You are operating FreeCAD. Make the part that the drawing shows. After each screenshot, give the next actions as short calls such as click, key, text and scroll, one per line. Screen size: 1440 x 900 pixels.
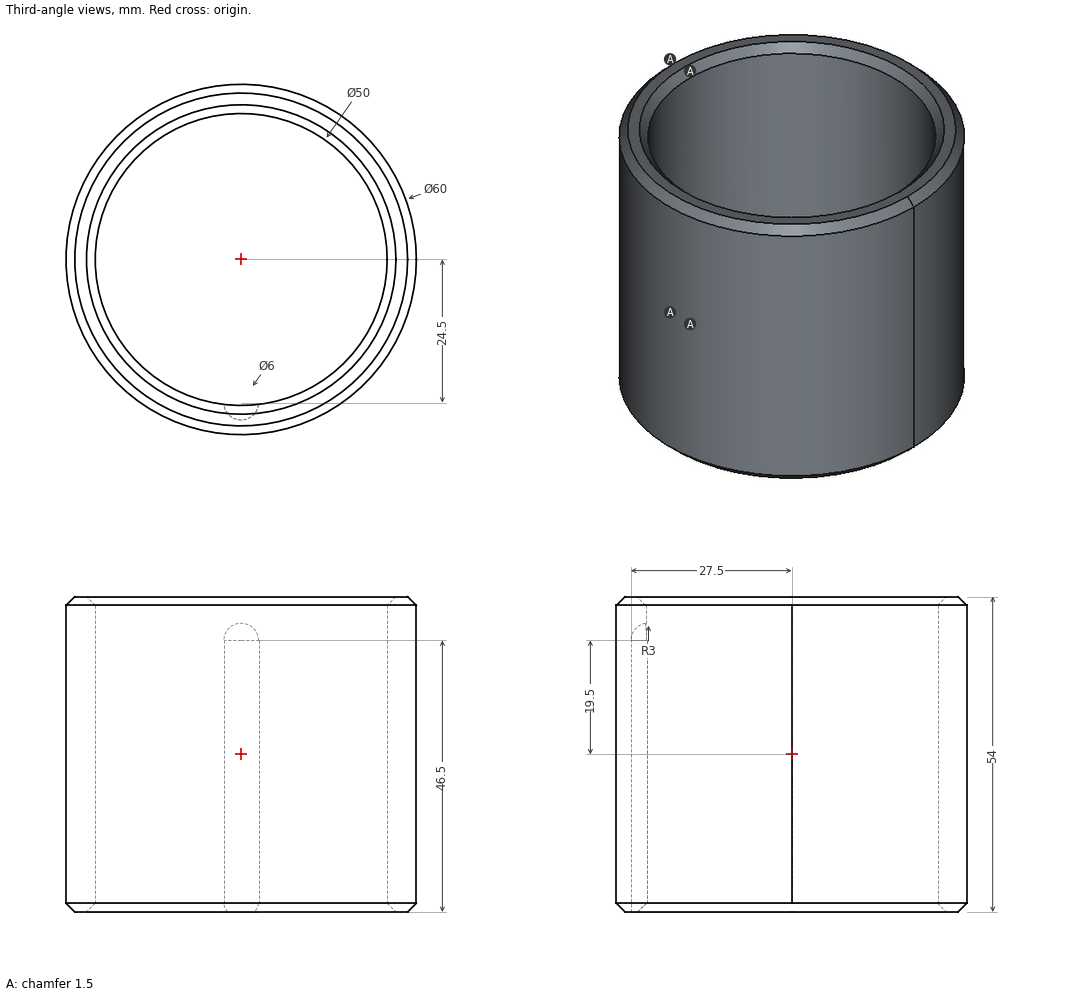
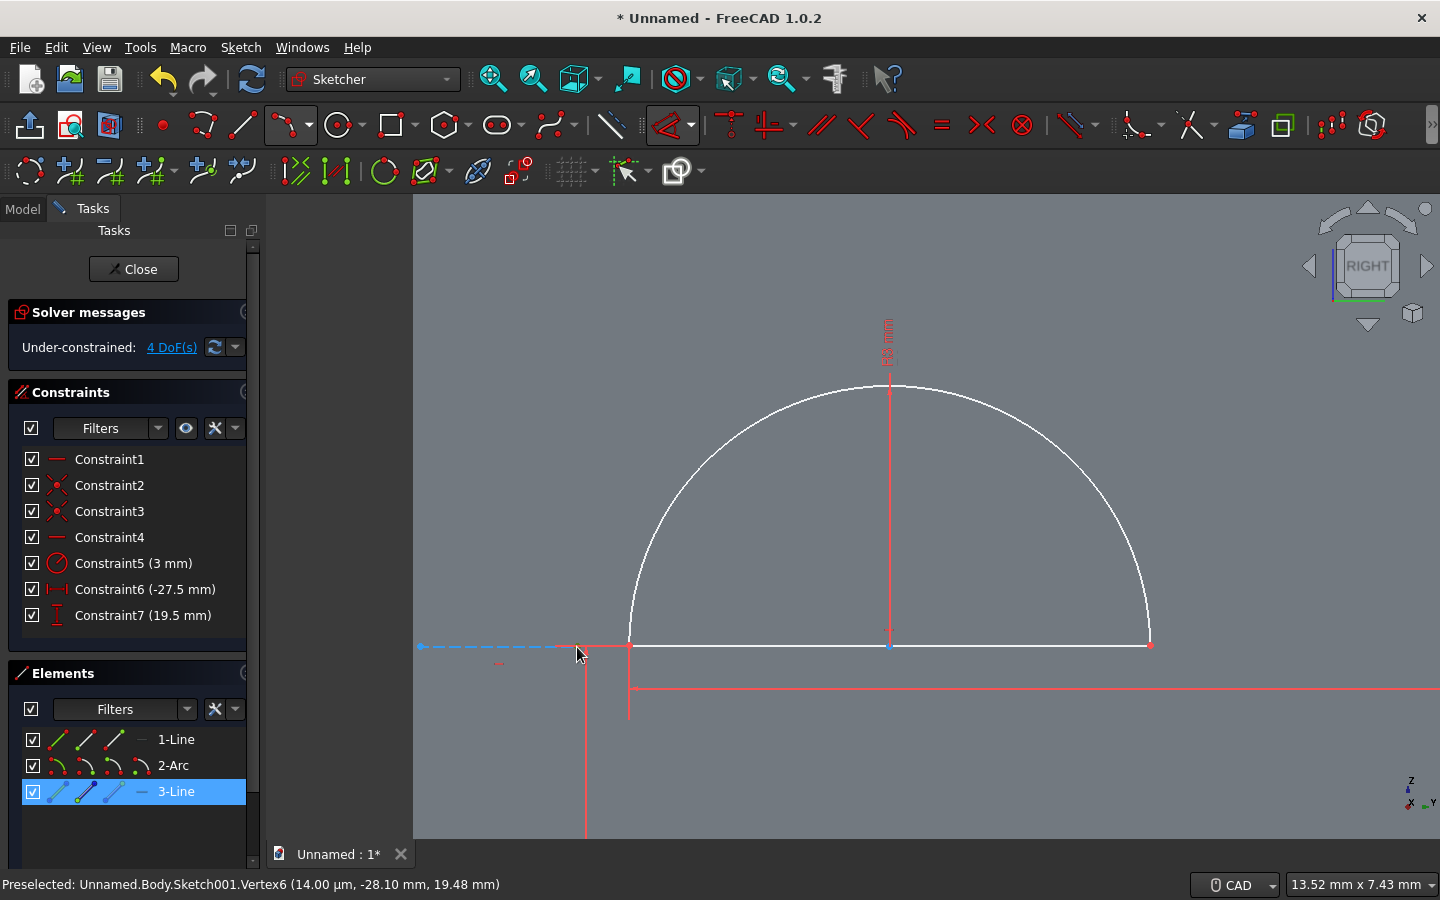
key(i)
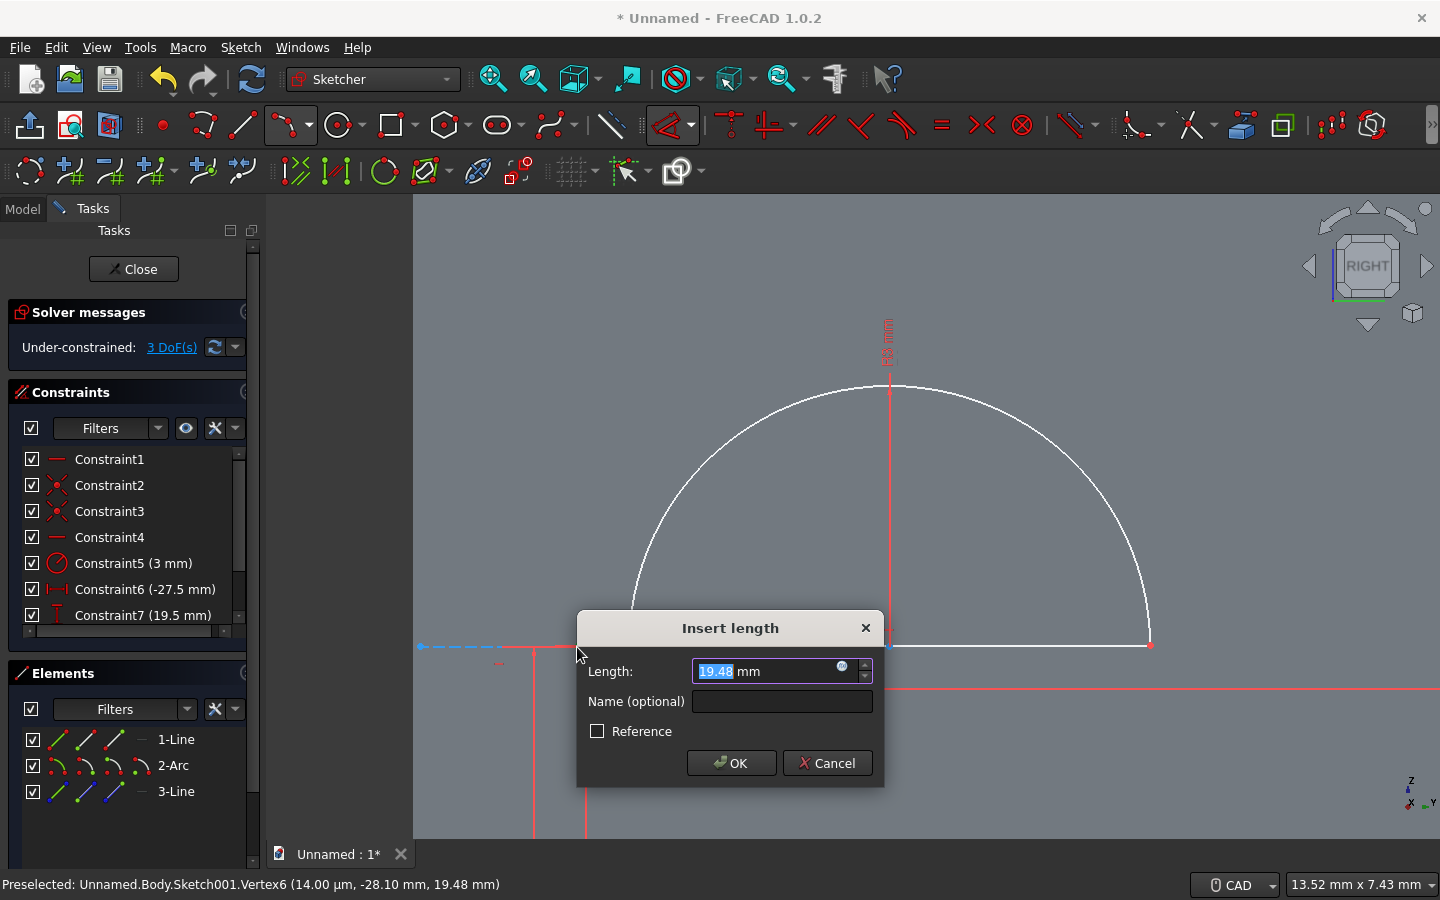
text(19.5)
key(Return)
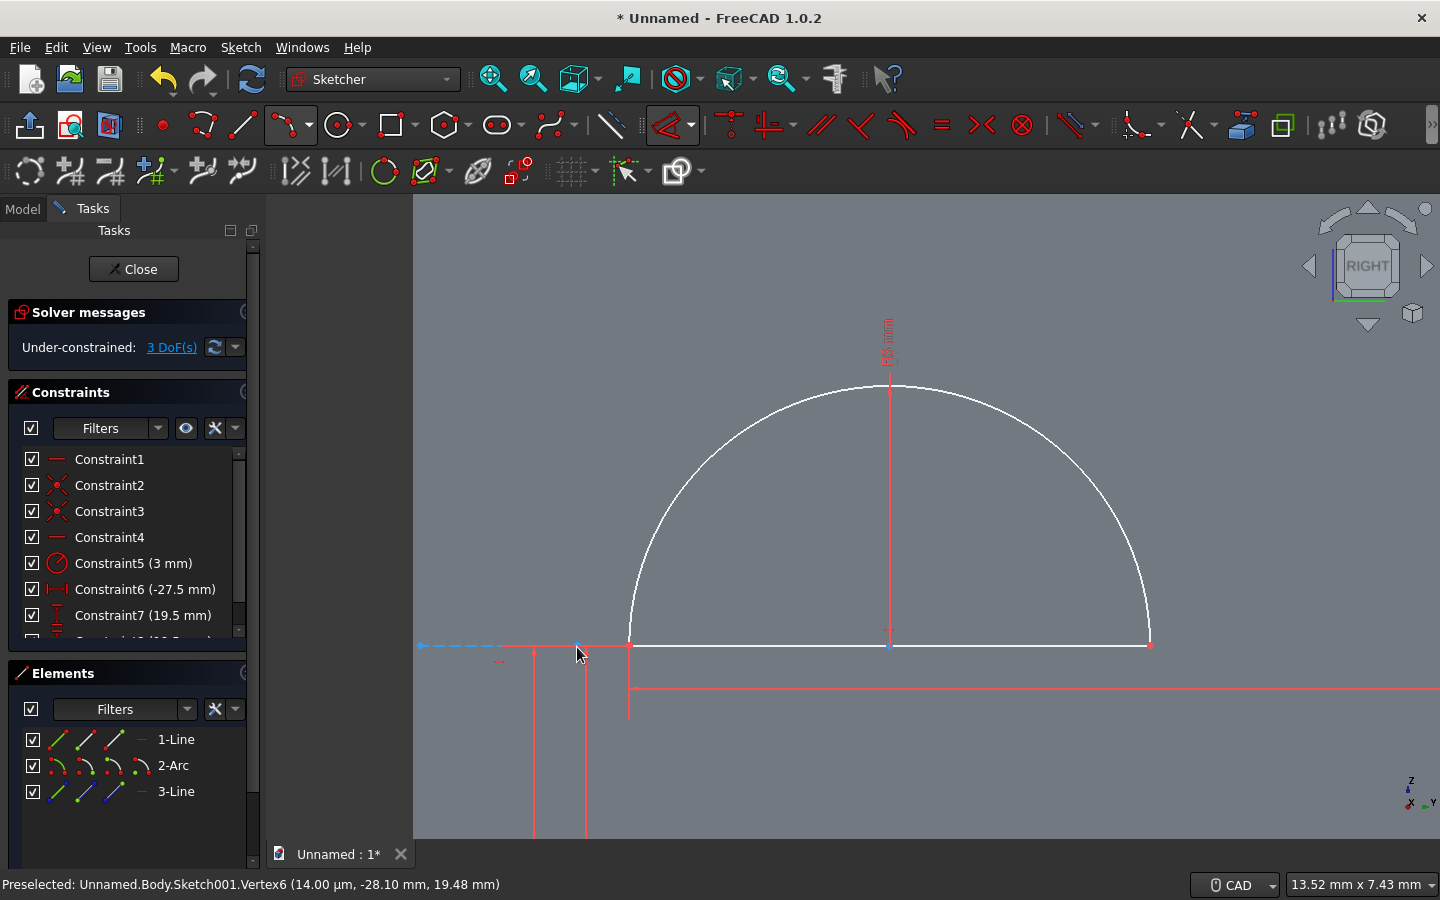
click(890, 647)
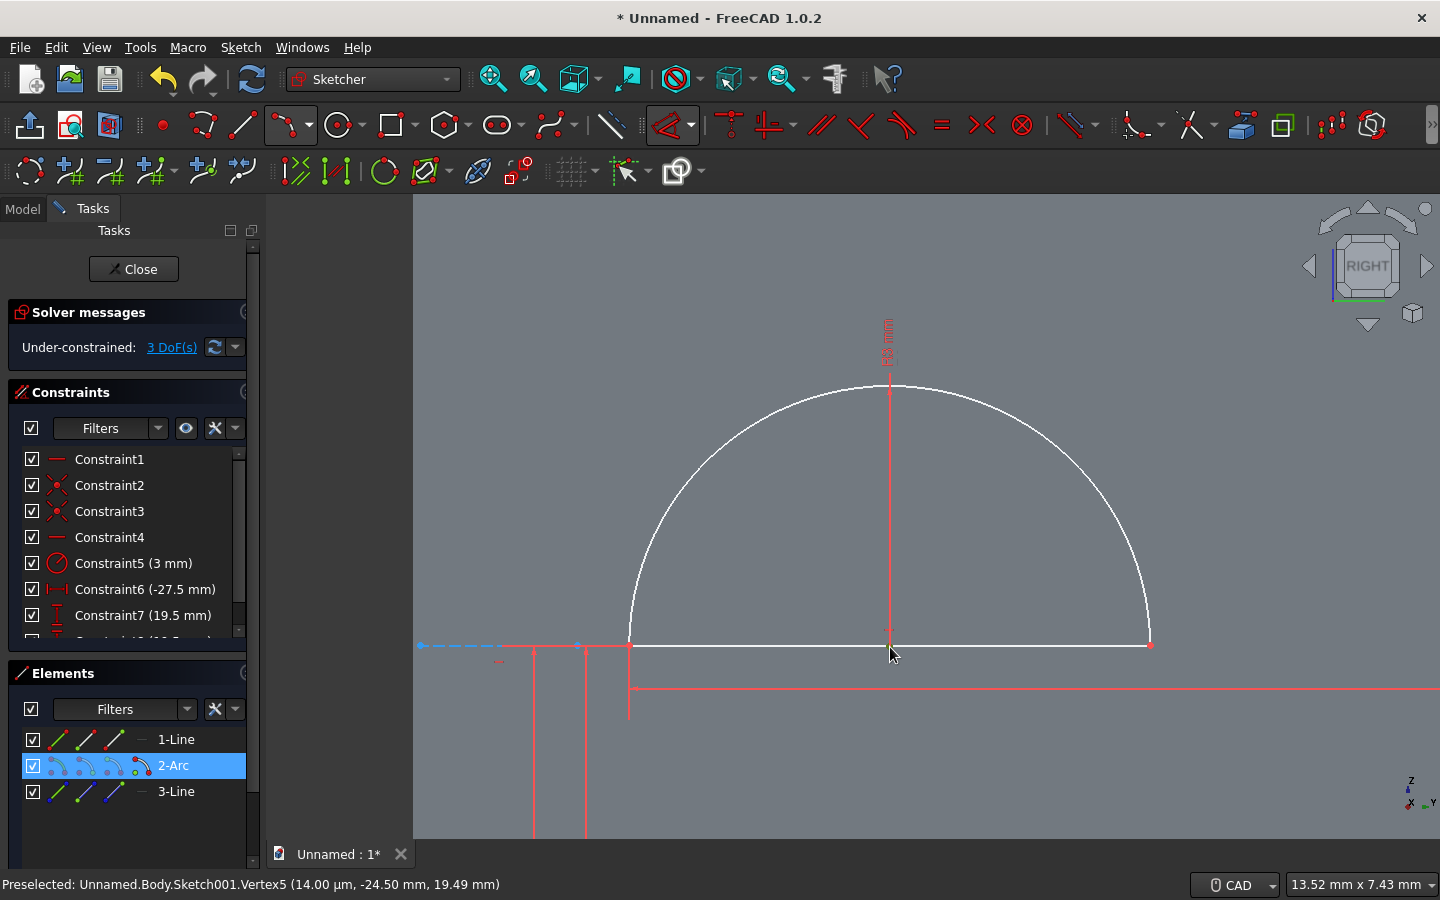
key(i)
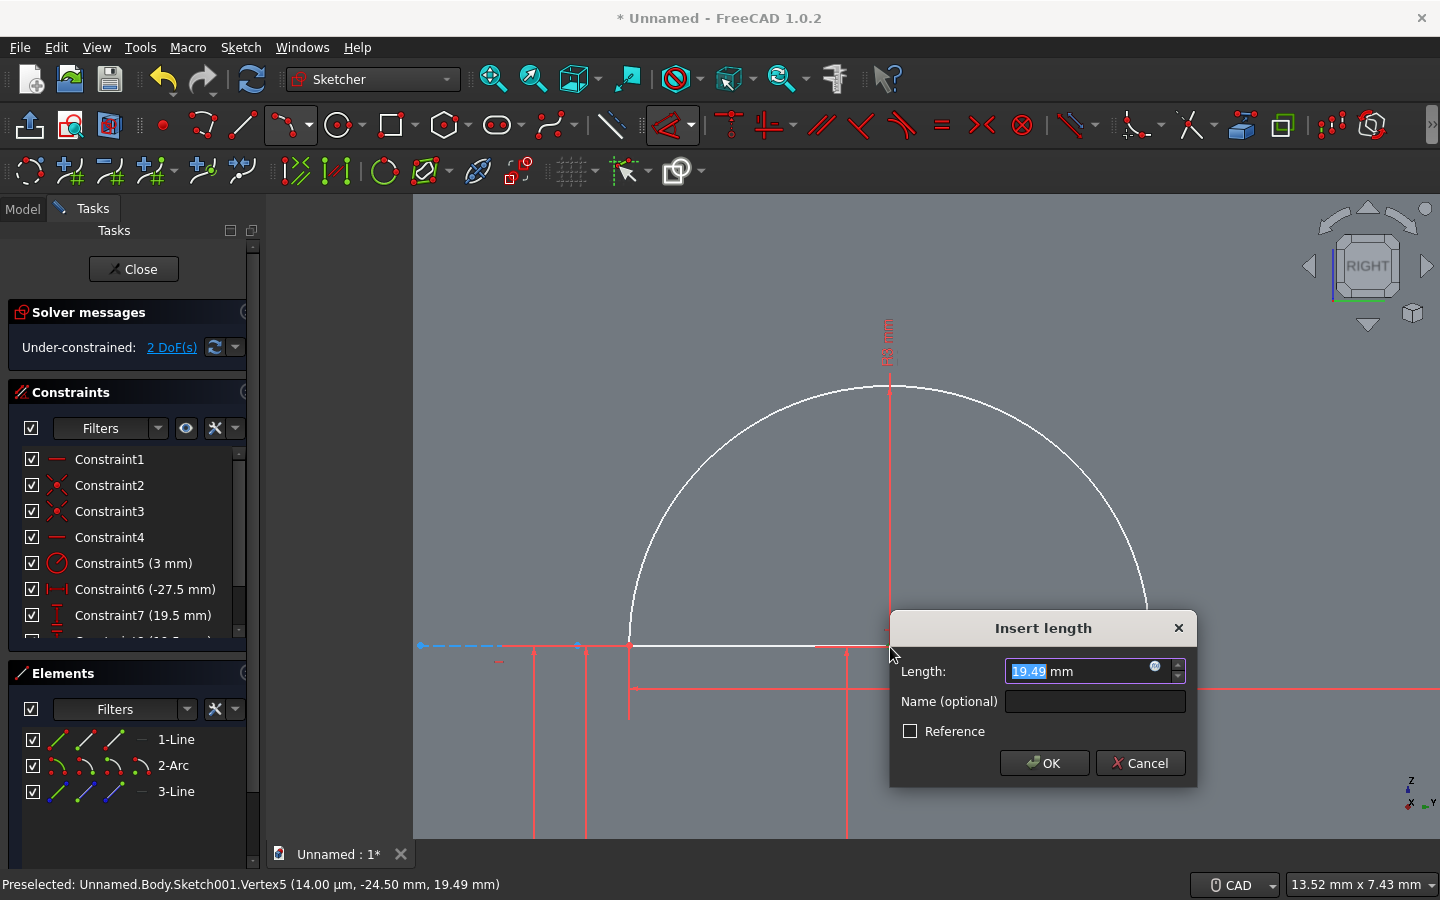
text(19.5)
key(Return)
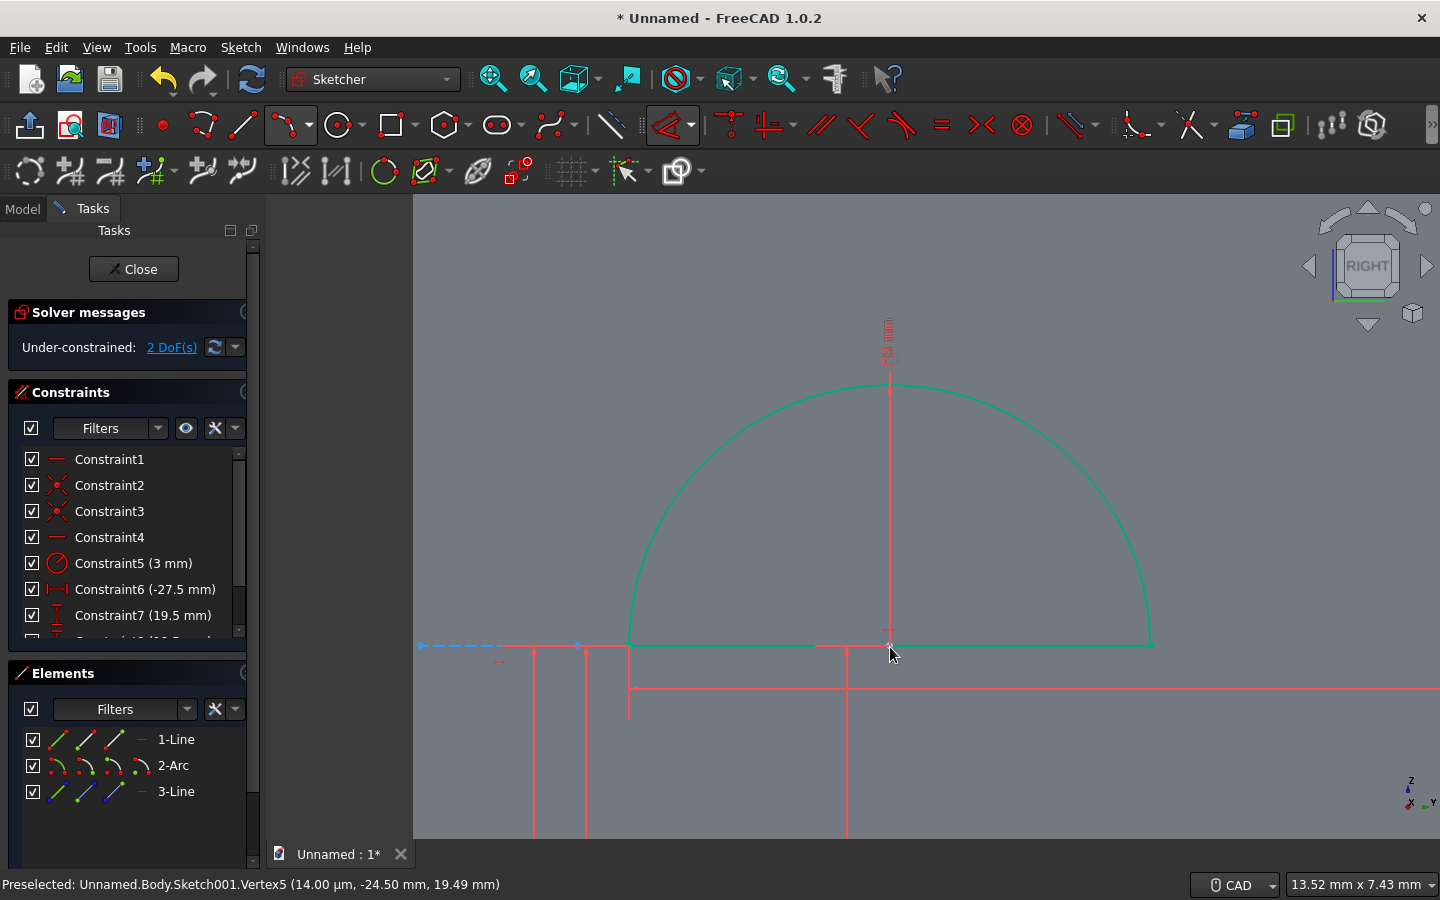
click(134, 269)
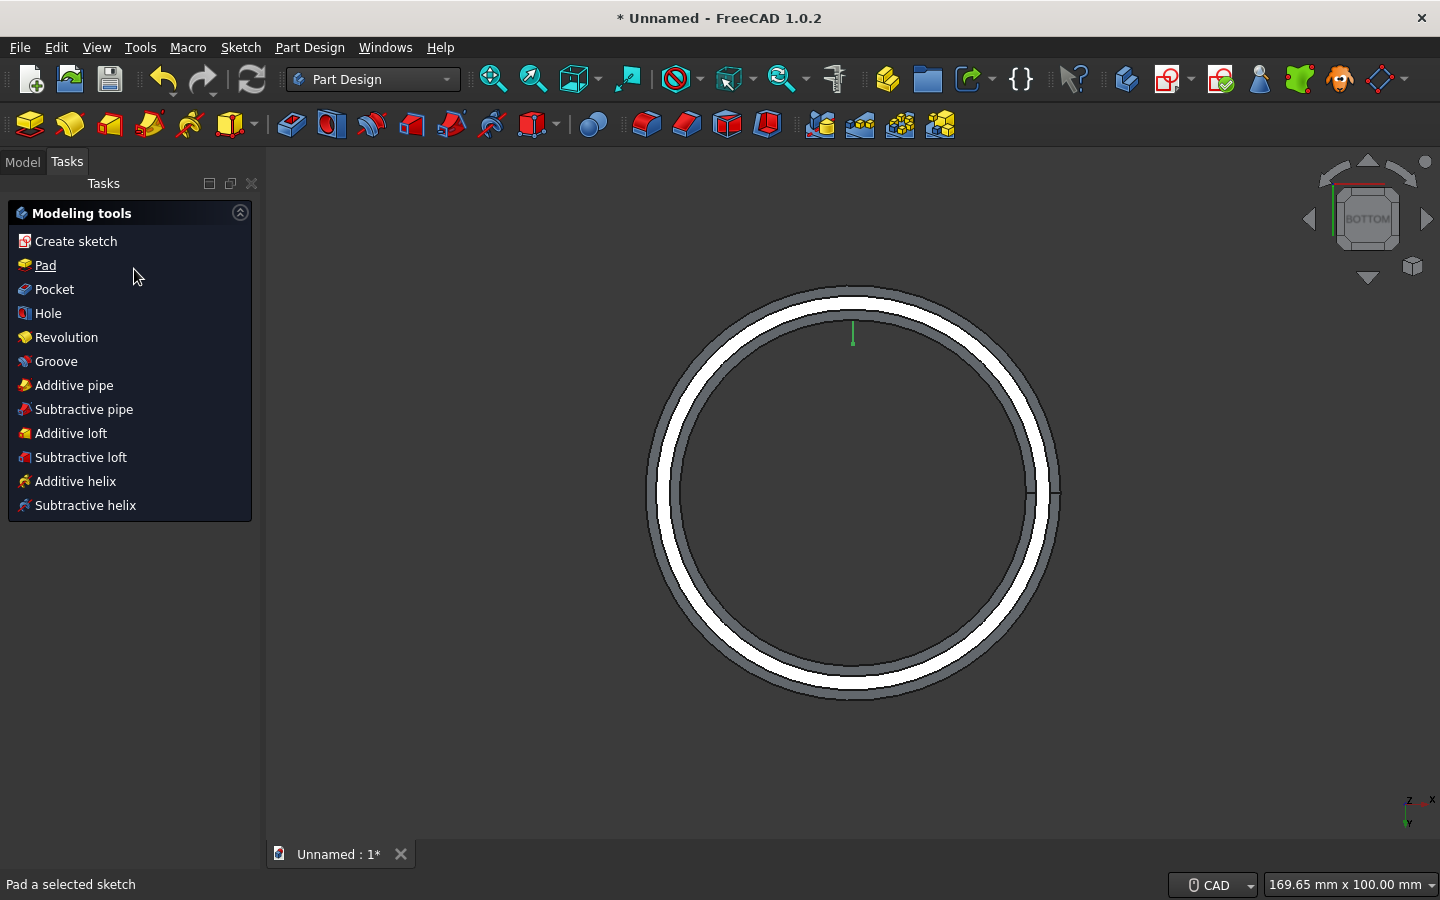
click(372, 124)